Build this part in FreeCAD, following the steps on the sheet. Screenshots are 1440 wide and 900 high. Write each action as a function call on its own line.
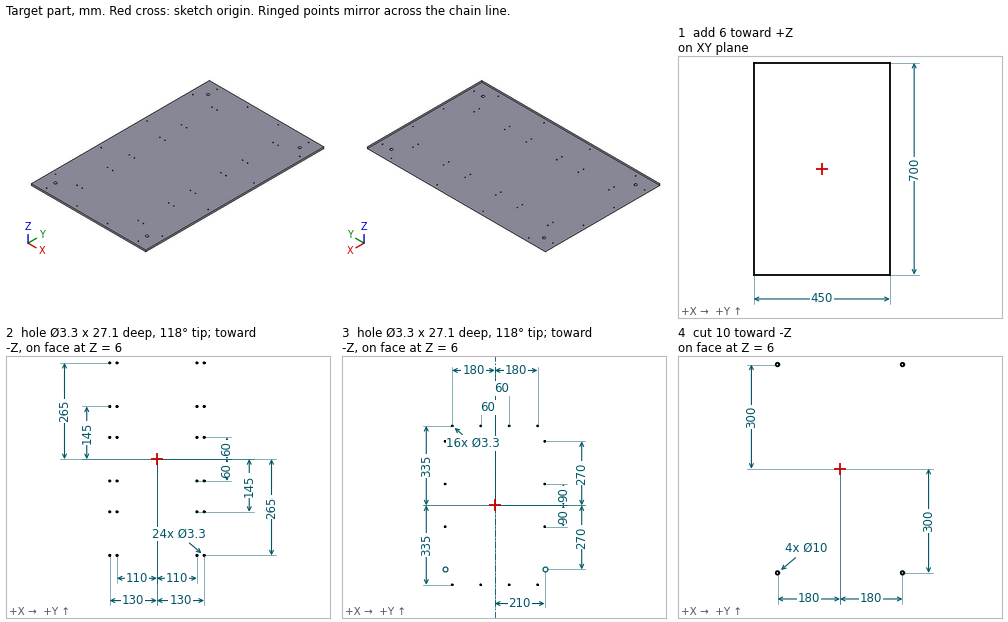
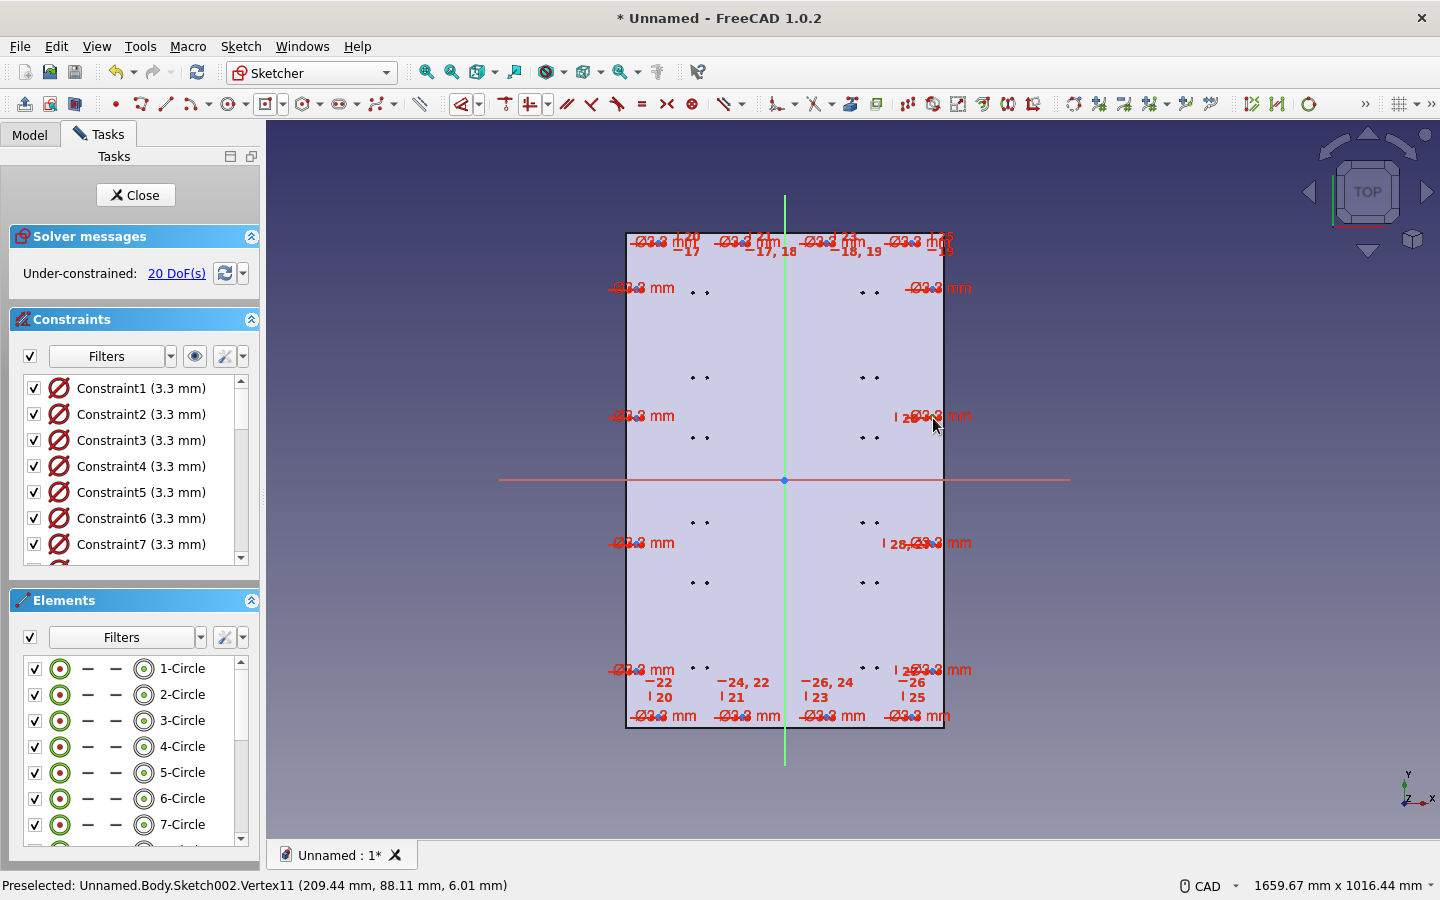
click(933, 290)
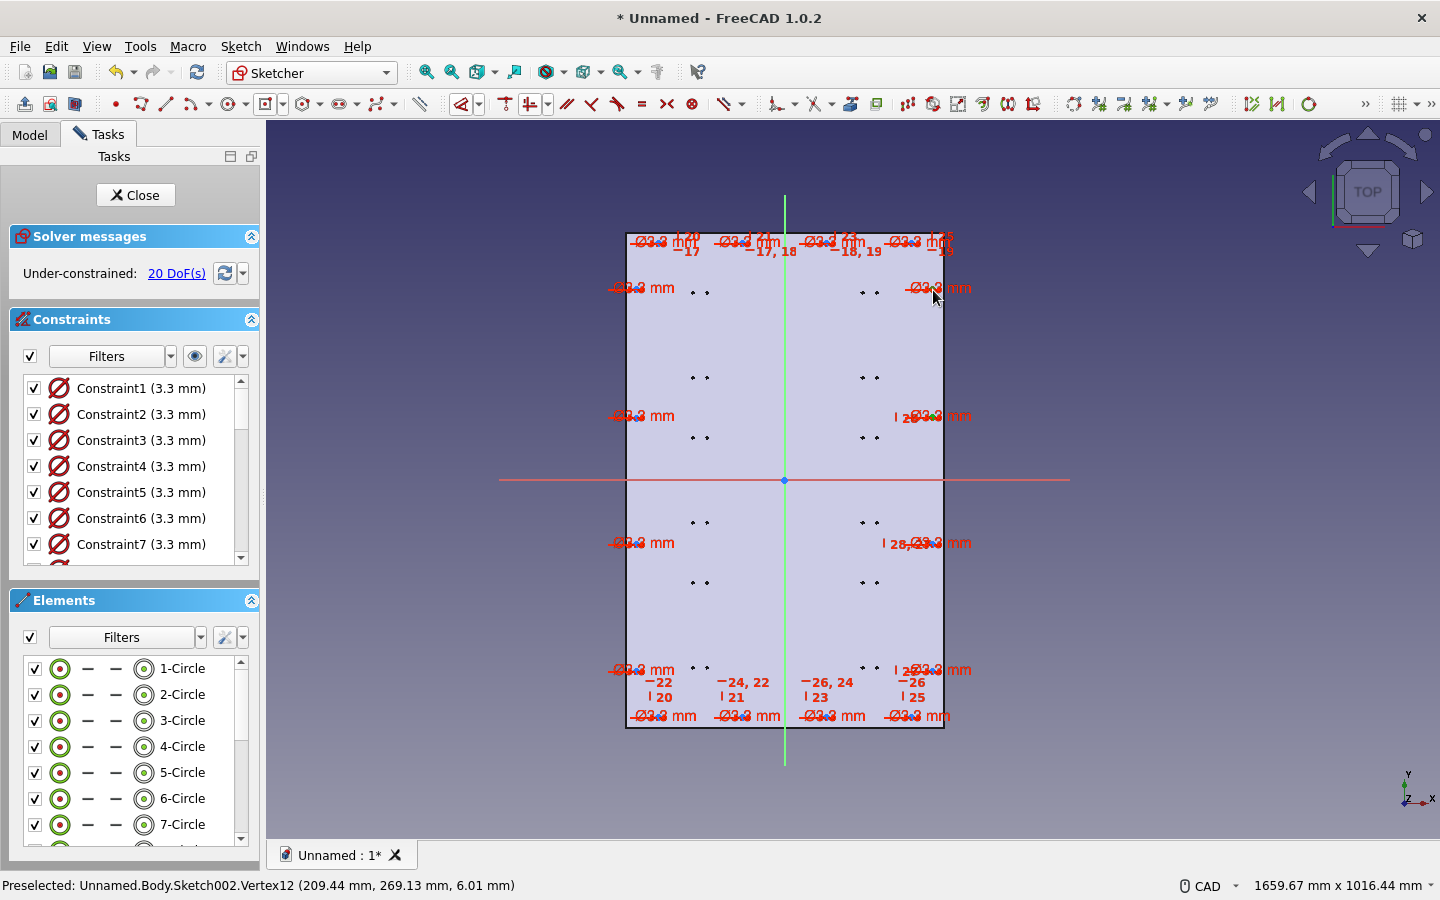
click(548, 104)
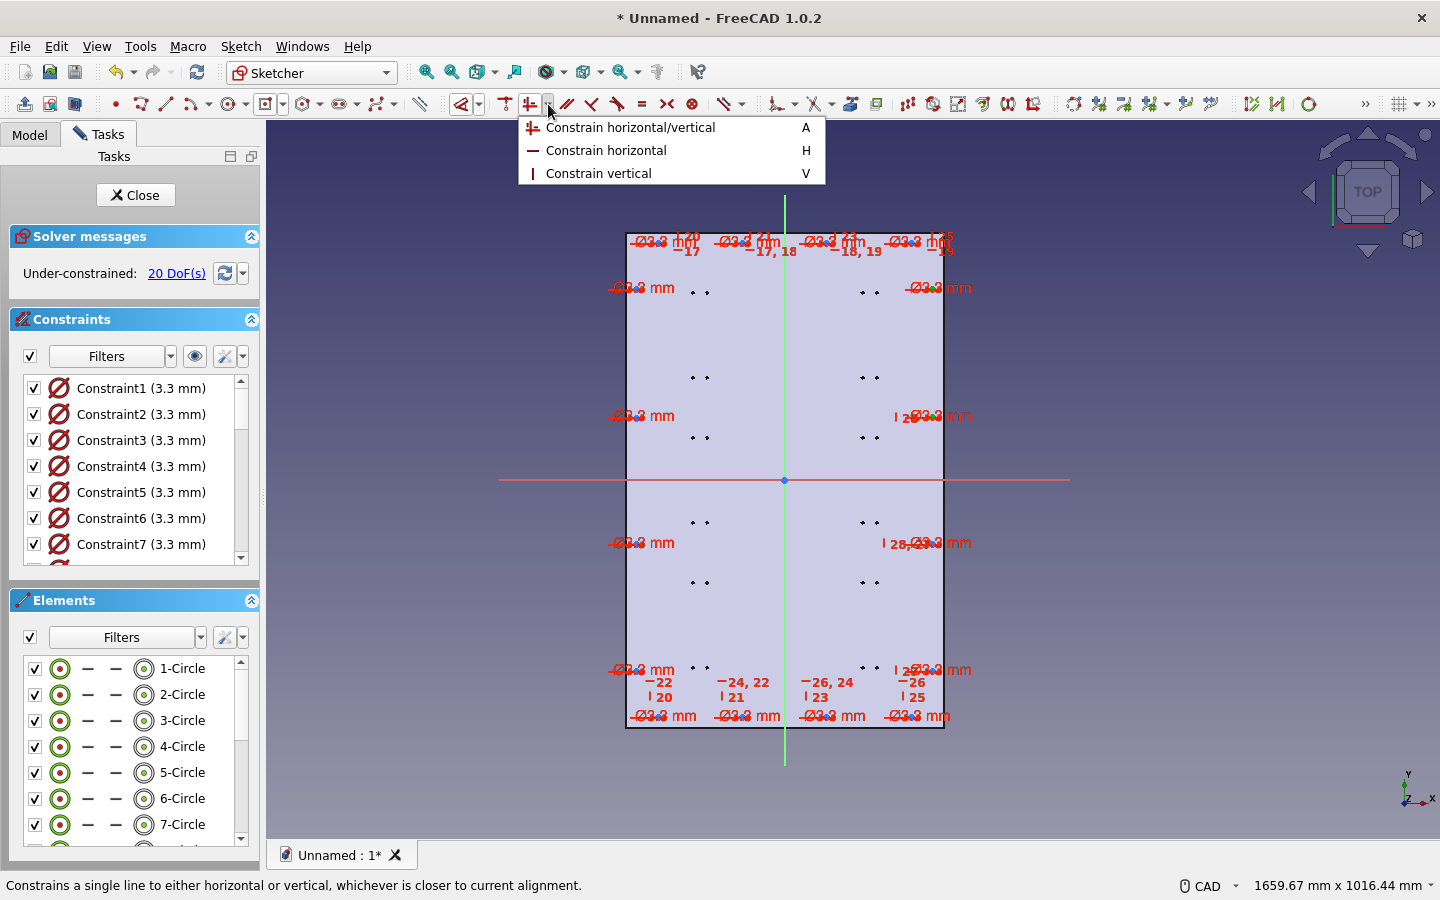
click(672, 174)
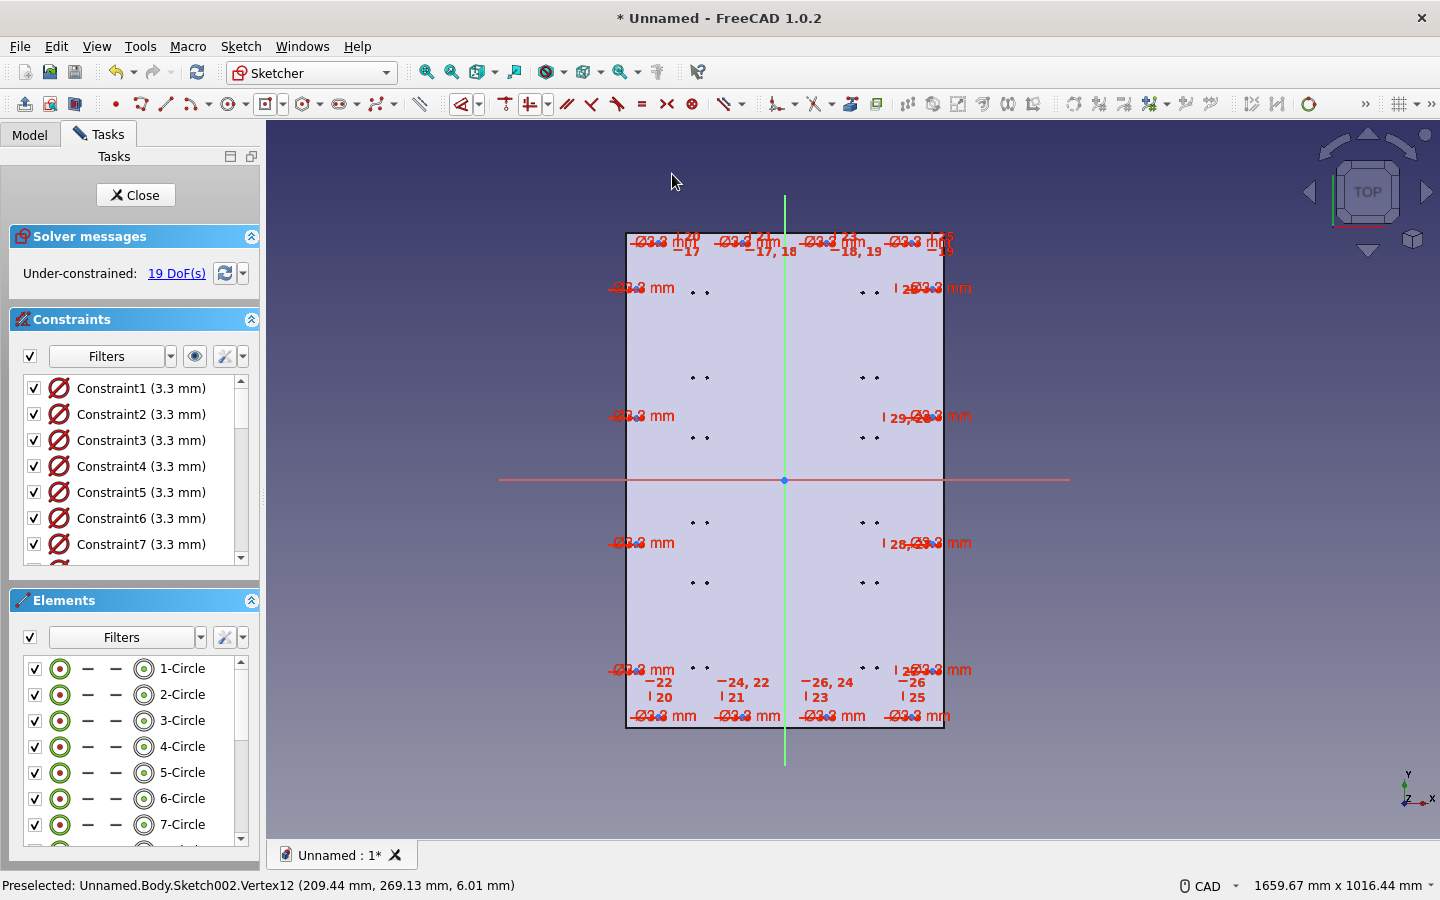
click(933, 290)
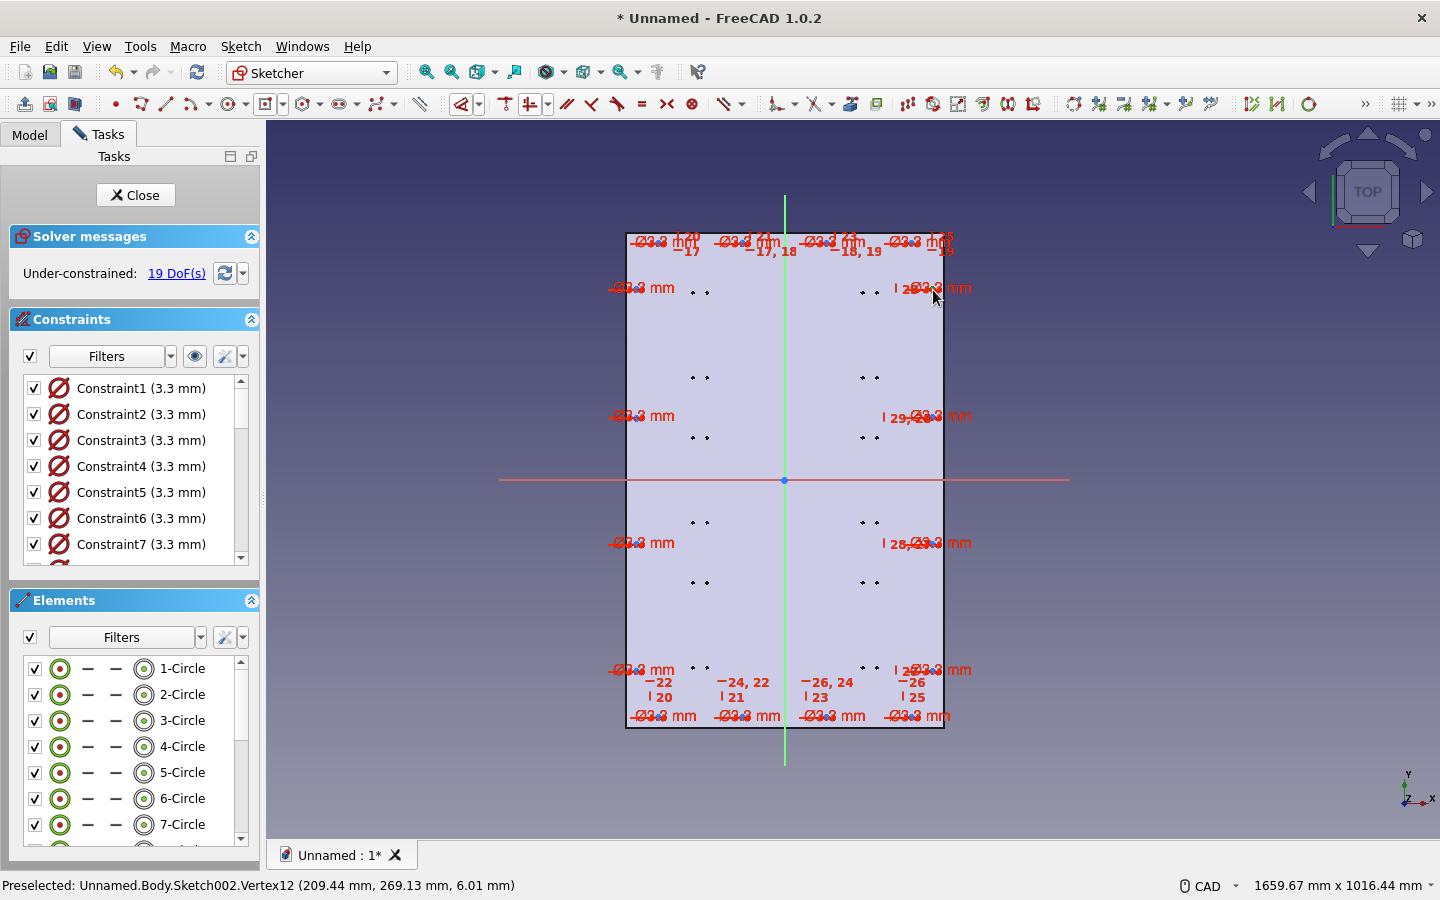
click(636, 290)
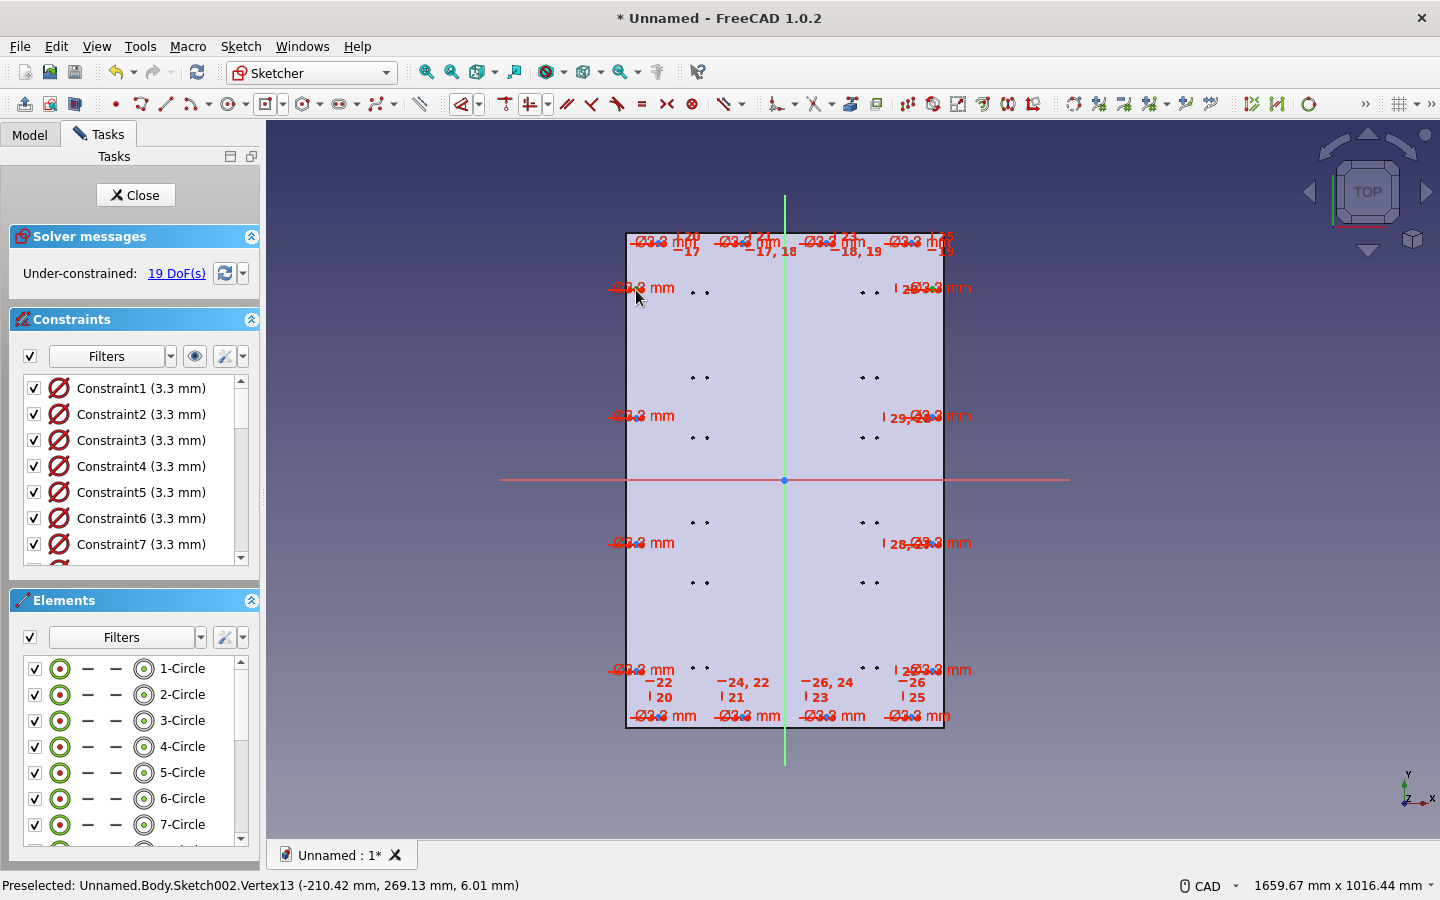
key(h)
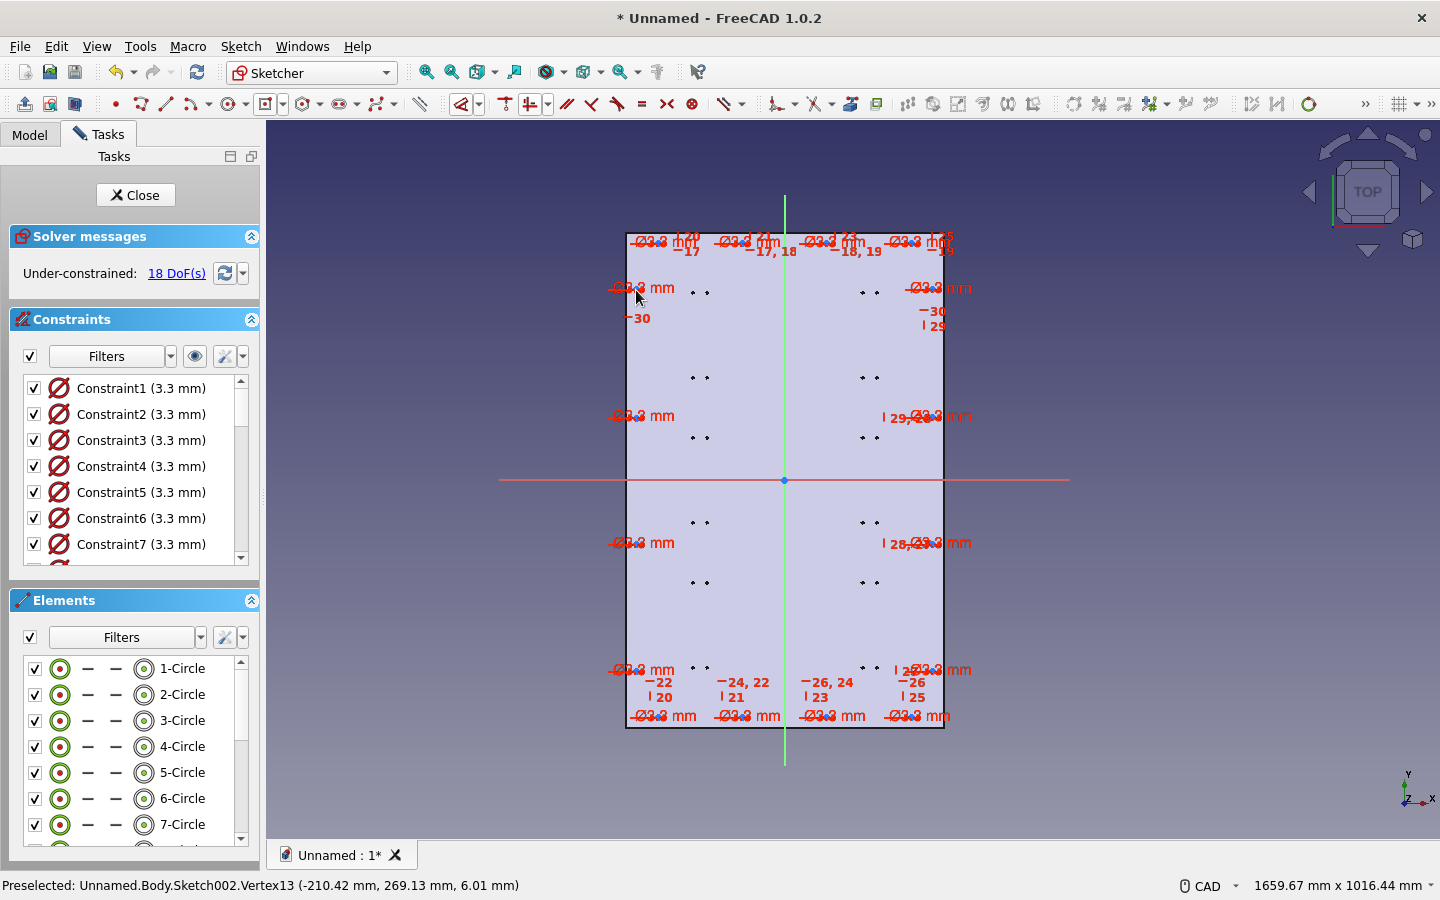
click(636, 290)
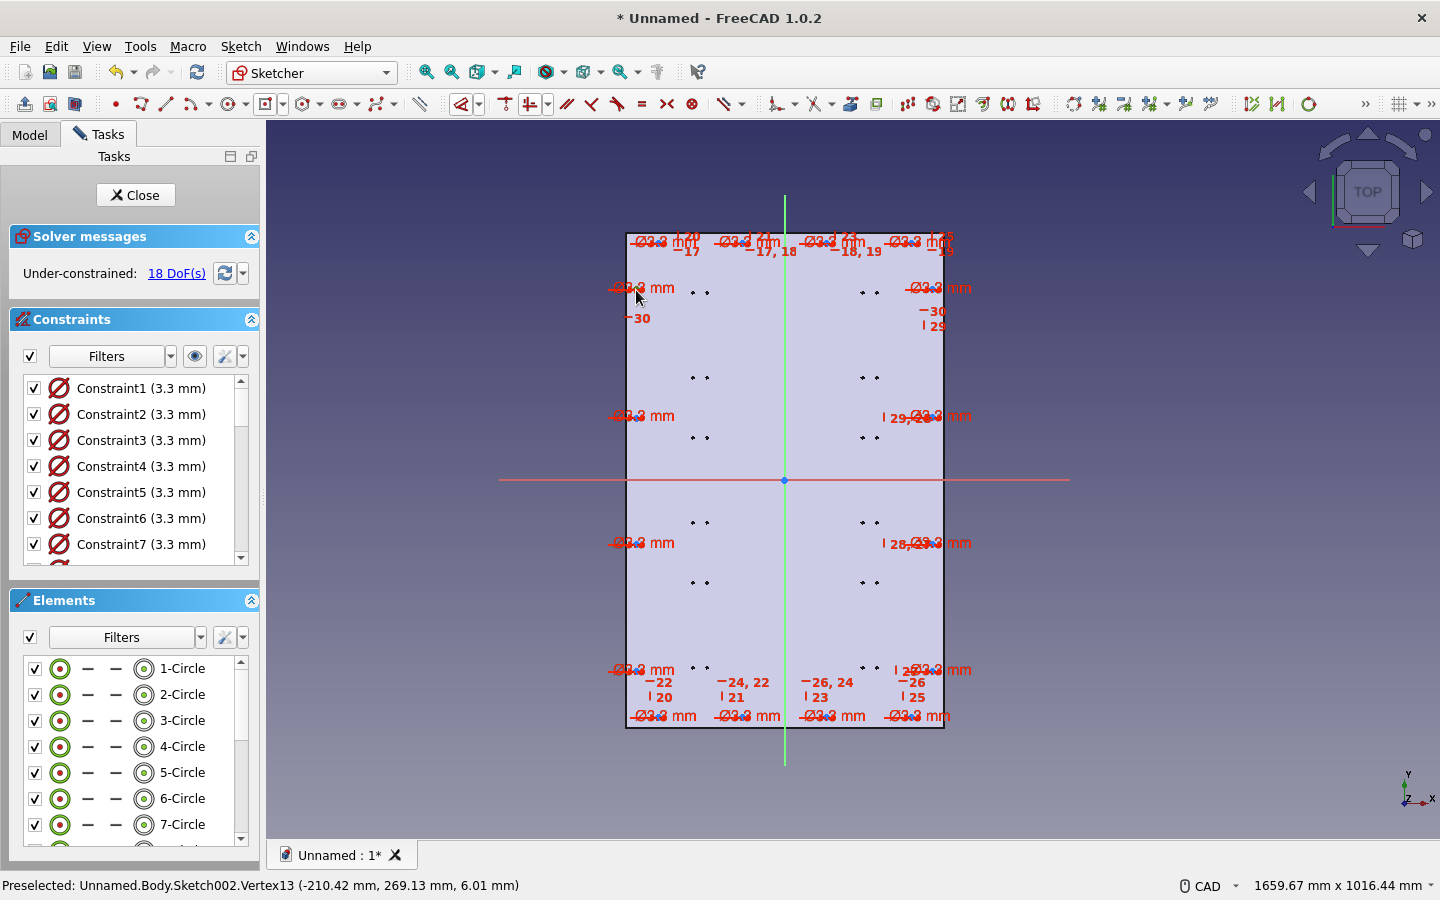
click(636, 418)